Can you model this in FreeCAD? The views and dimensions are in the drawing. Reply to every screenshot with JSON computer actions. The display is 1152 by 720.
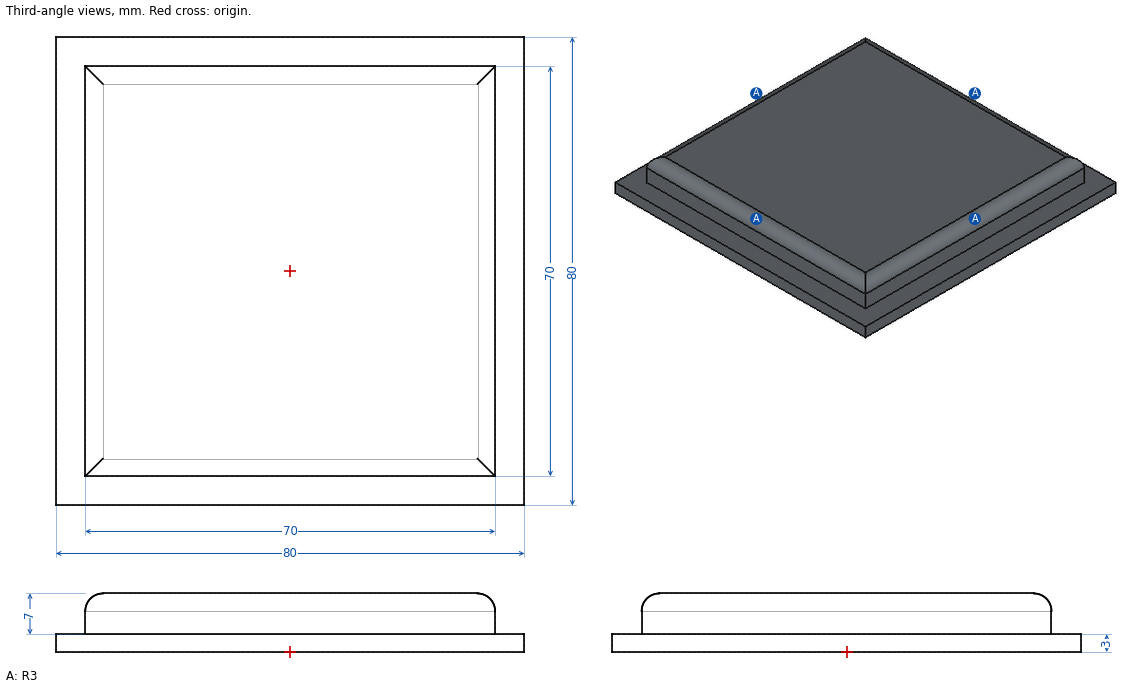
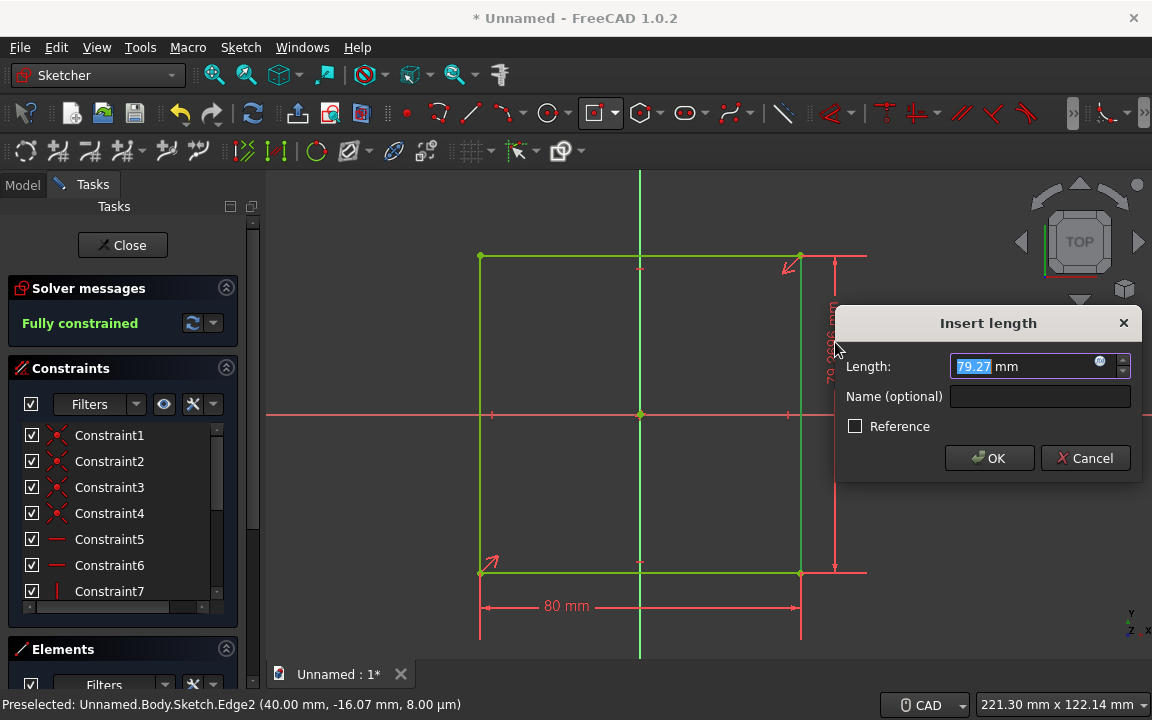
{"action": "type", "text": "80"}
{"action": "key", "text": "Return"}
{"action": "key", "text": "Escape"}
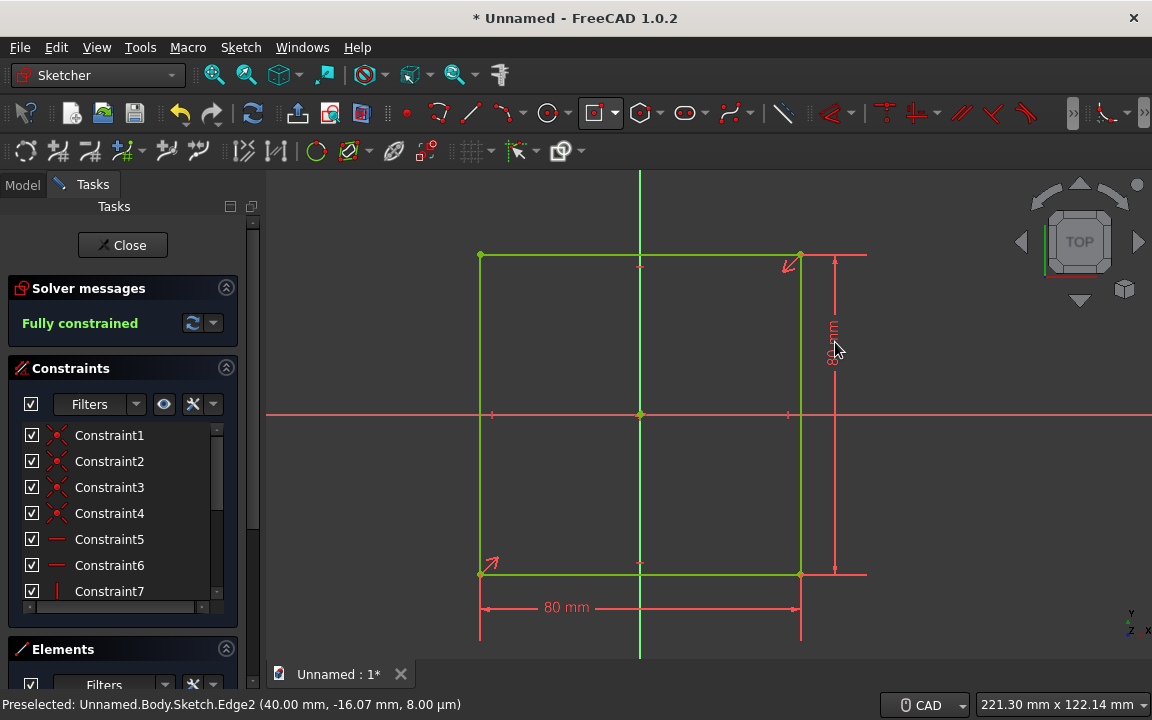
{"action": "left_click", "coordinate": [123, 245]}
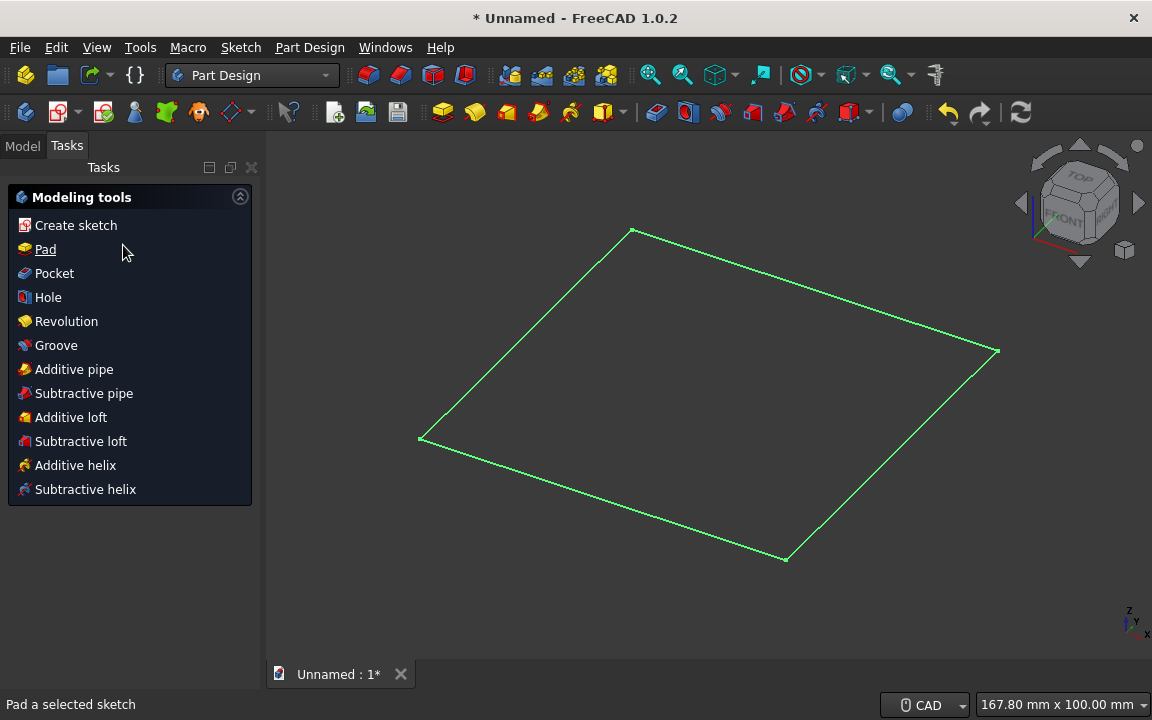
{"action": "left_click", "coordinate": [444, 112]}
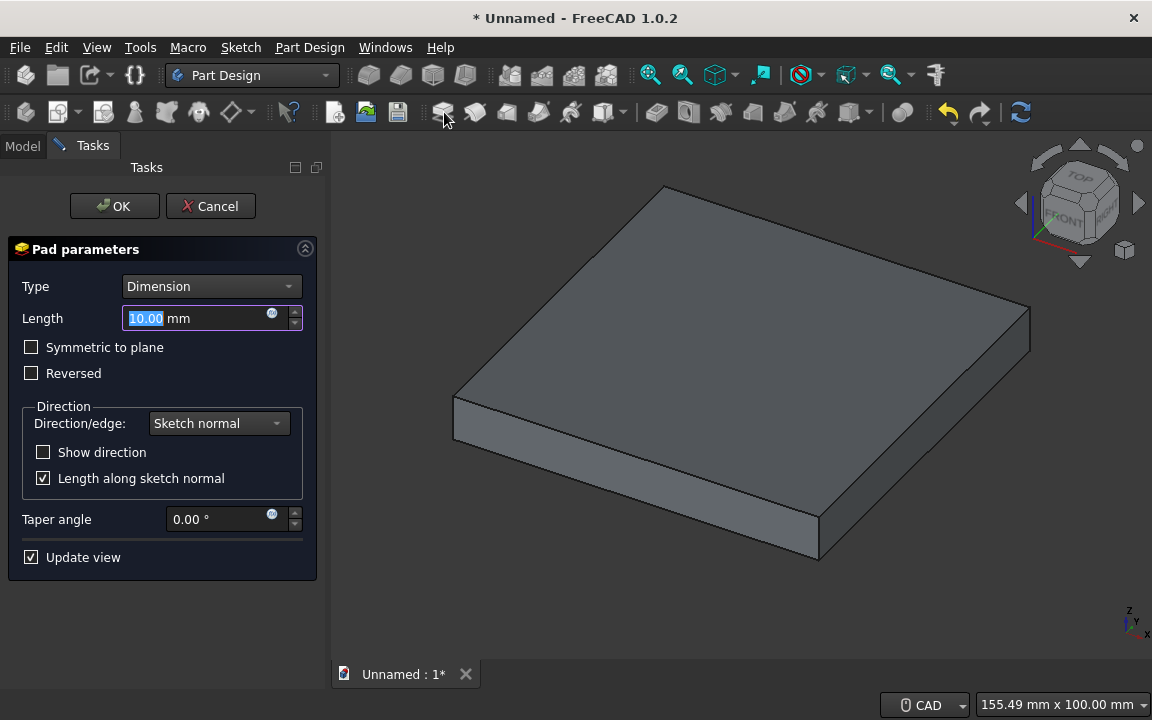
{"action": "type", "text": "3"}
{"action": "key", "text": "Tab"}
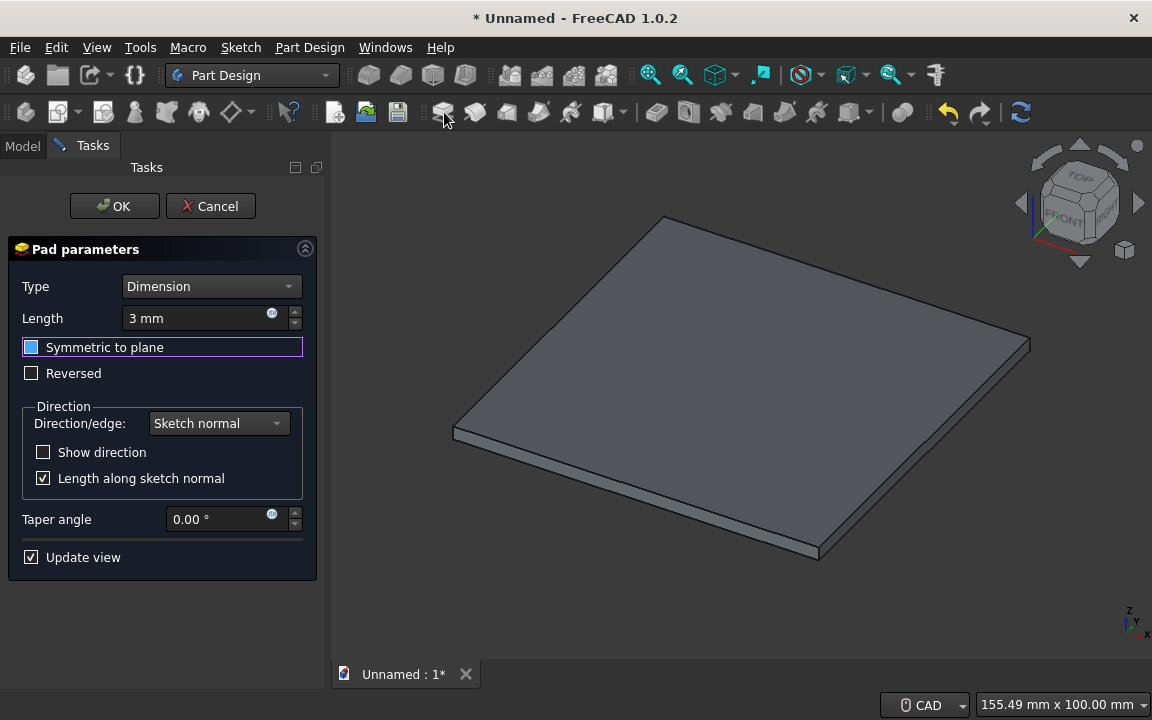
{"action": "left_click", "coordinate": [115, 206]}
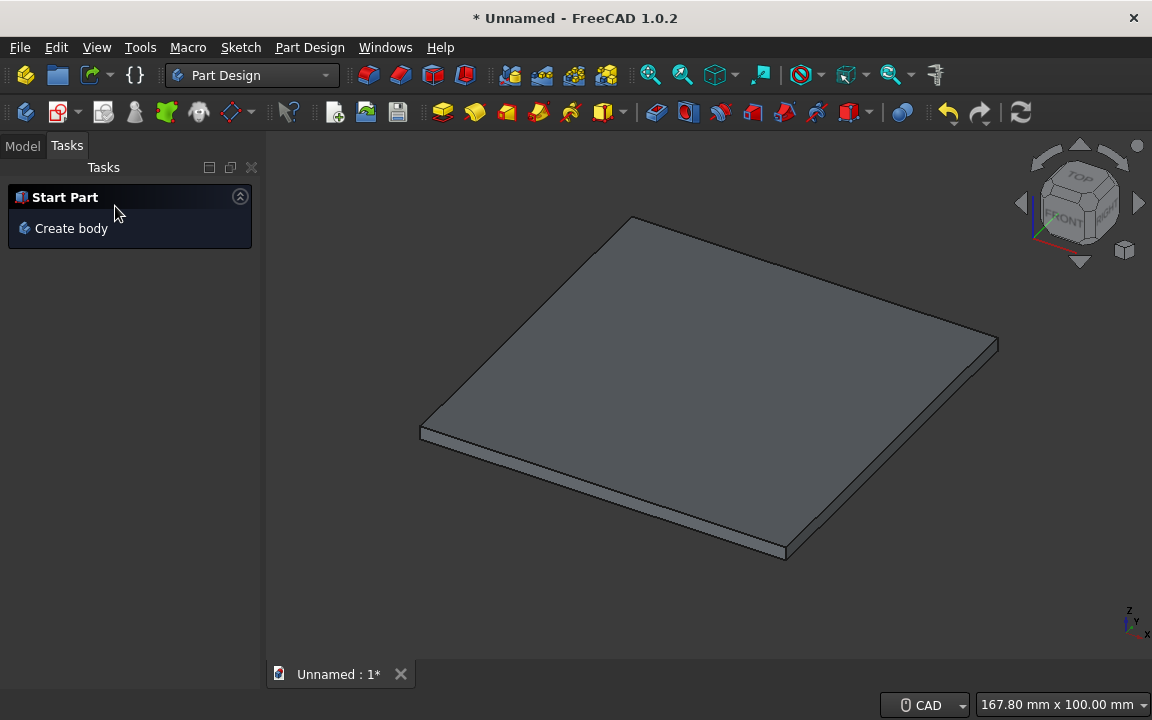
{"action": "left_click", "coordinate": [709, 381]}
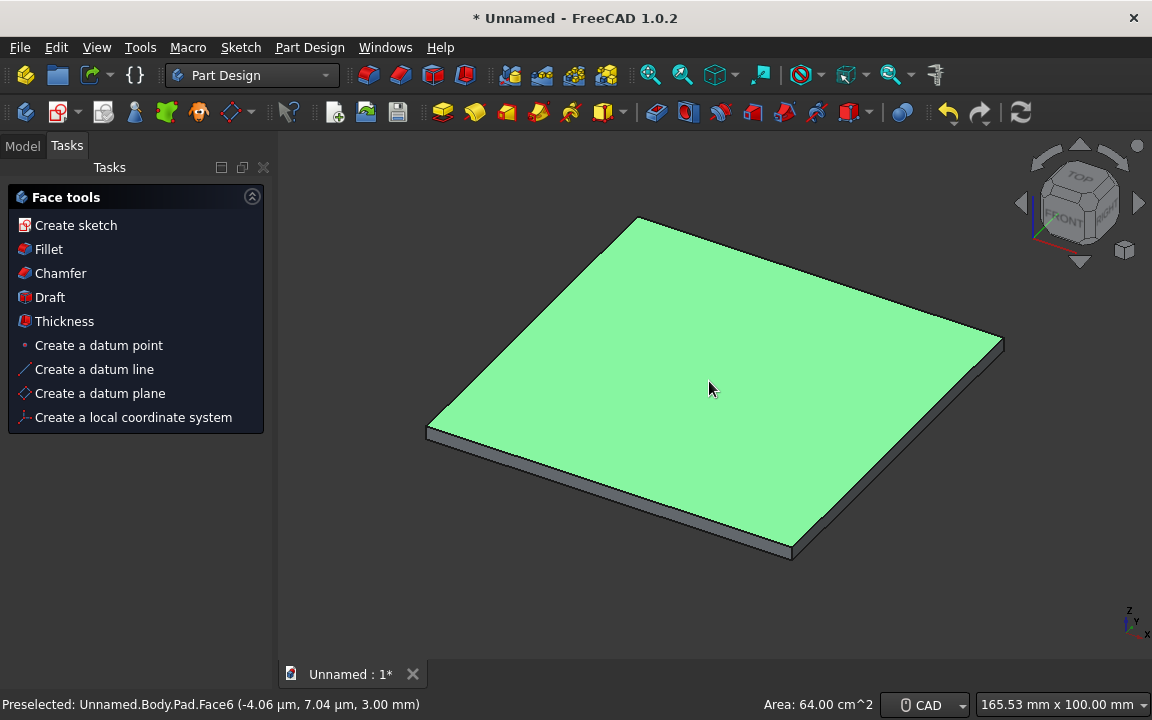
{"action": "left_click", "coordinate": [58, 112]}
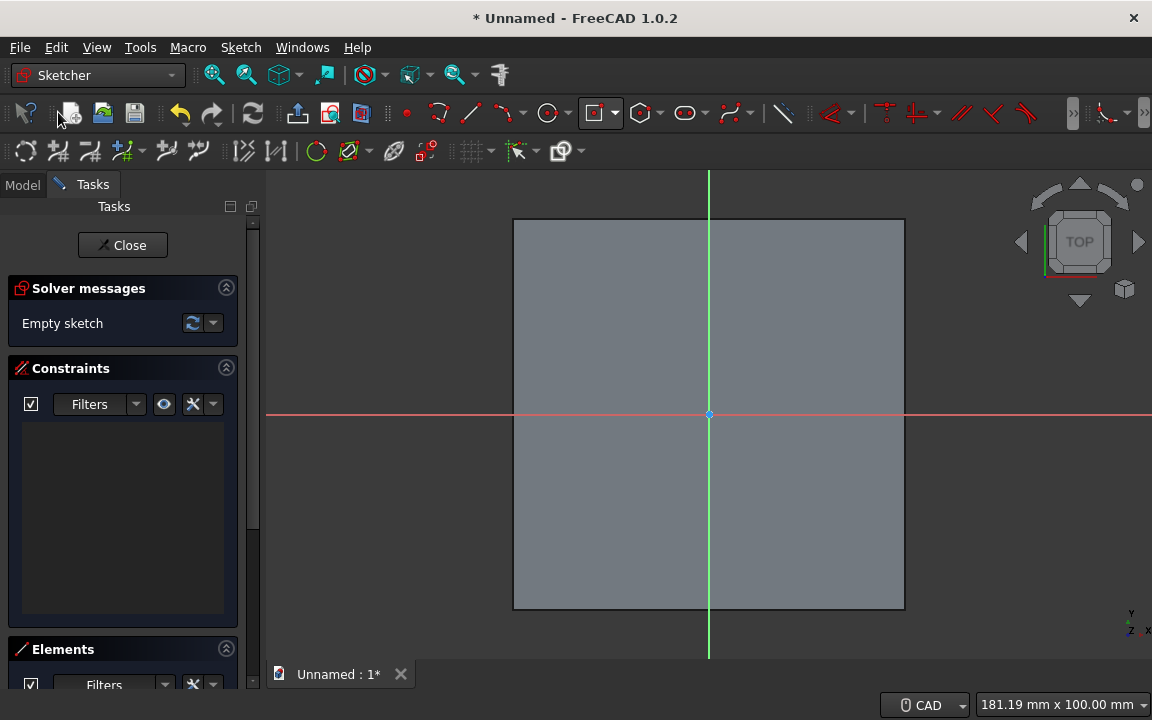
{"action": "left_click", "coordinate": [594, 114]}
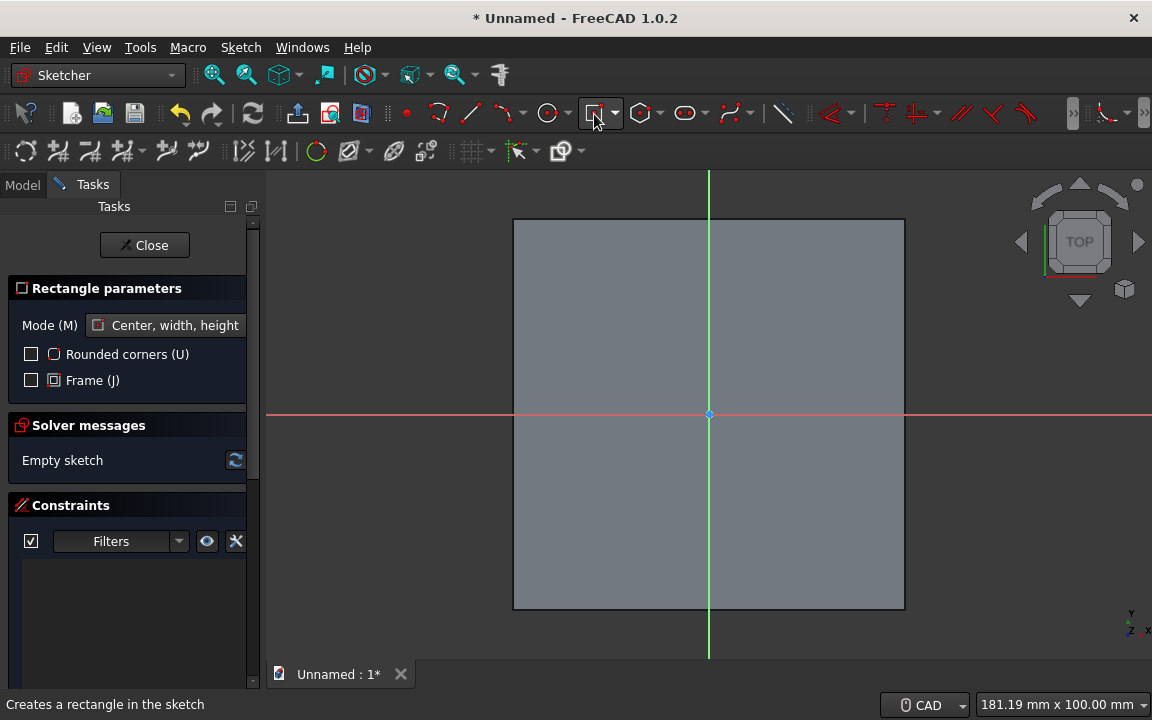
{"action": "left_click", "coordinate": [709, 414]}
{"action": "left_click", "coordinate": [880, 243]}
{"action": "key", "text": "Escape"}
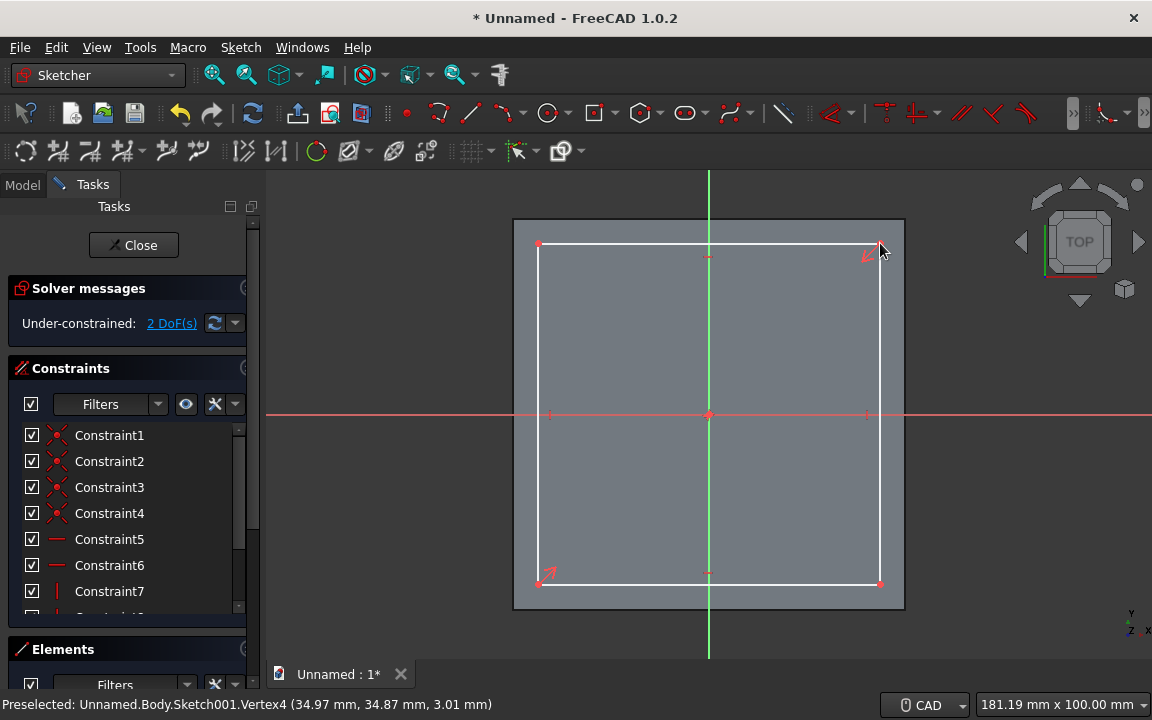
{"action": "left_click", "coordinate": [830, 114]}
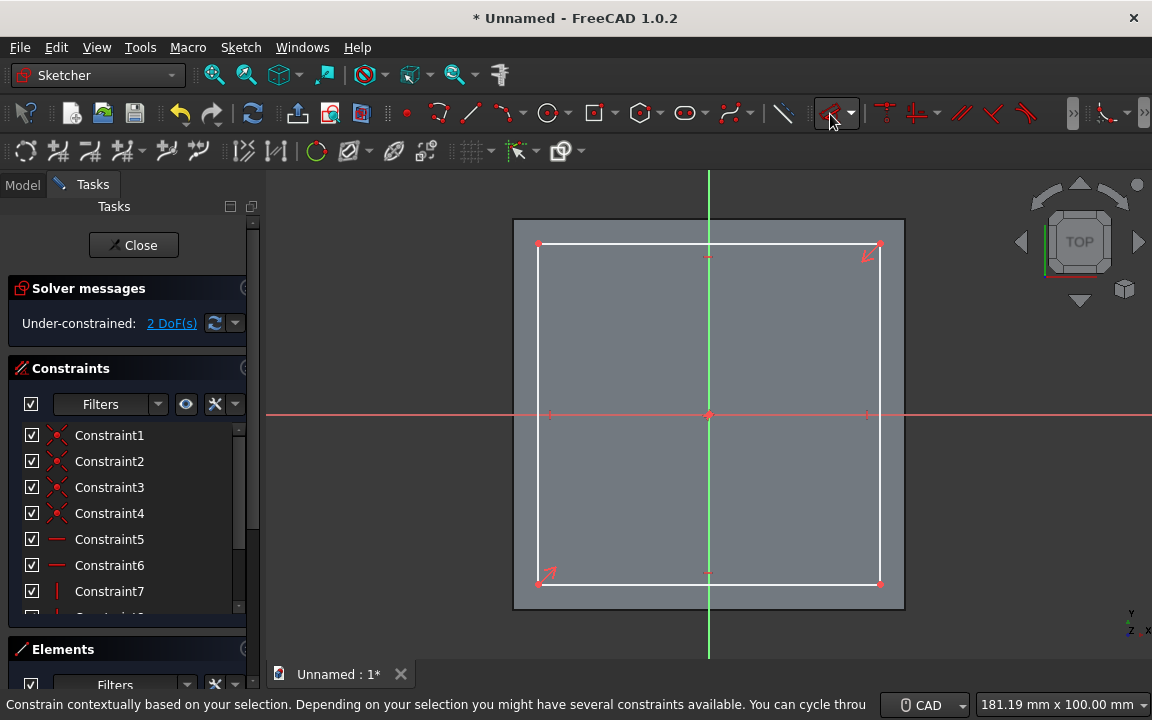
{"action": "left_click", "coordinate": [641, 585]}
{"action": "left_click", "coordinate": [630, 619]}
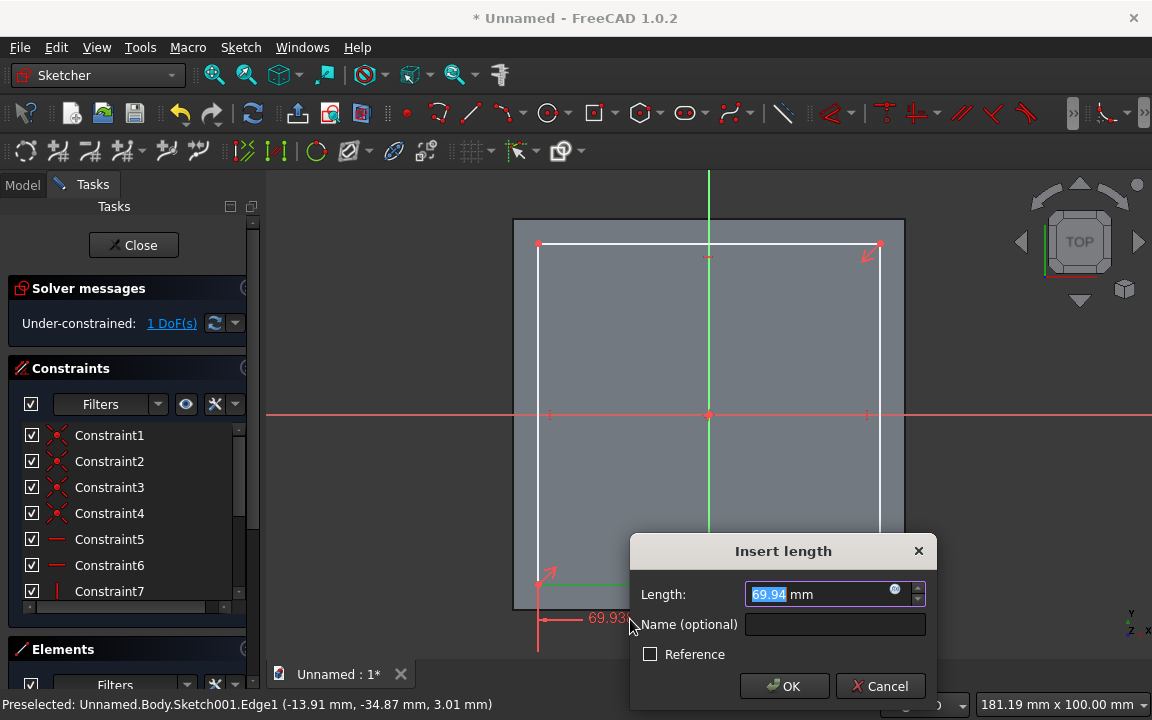
{"action": "type", "text": "70"}
{"action": "key", "text": "Return"}